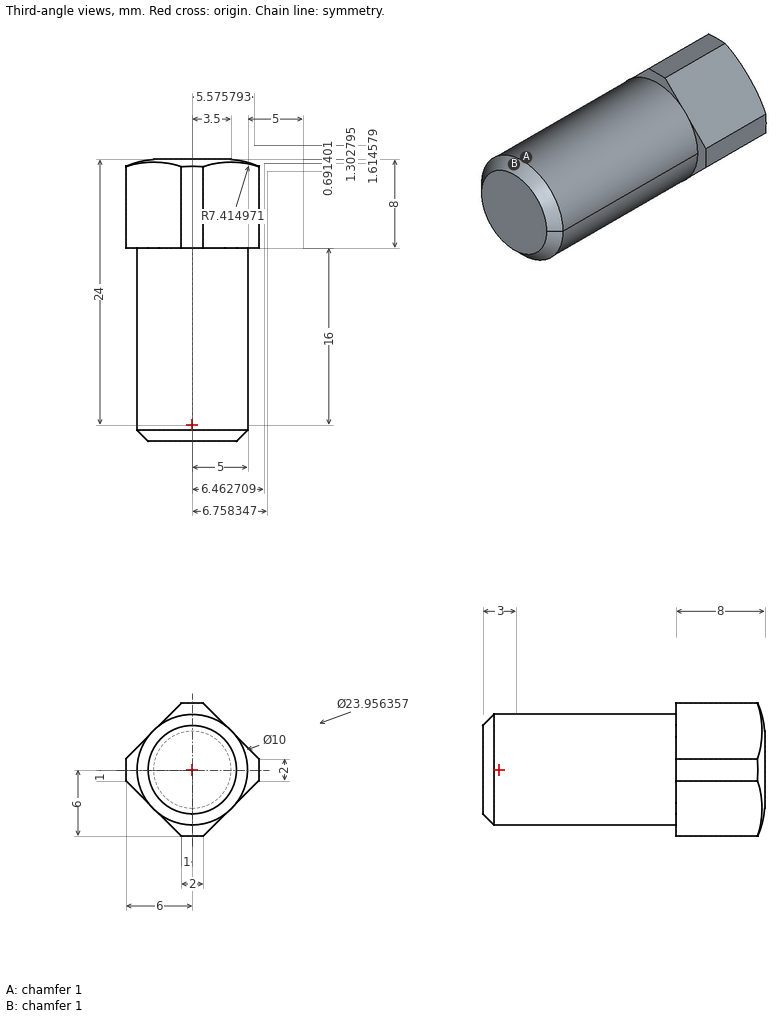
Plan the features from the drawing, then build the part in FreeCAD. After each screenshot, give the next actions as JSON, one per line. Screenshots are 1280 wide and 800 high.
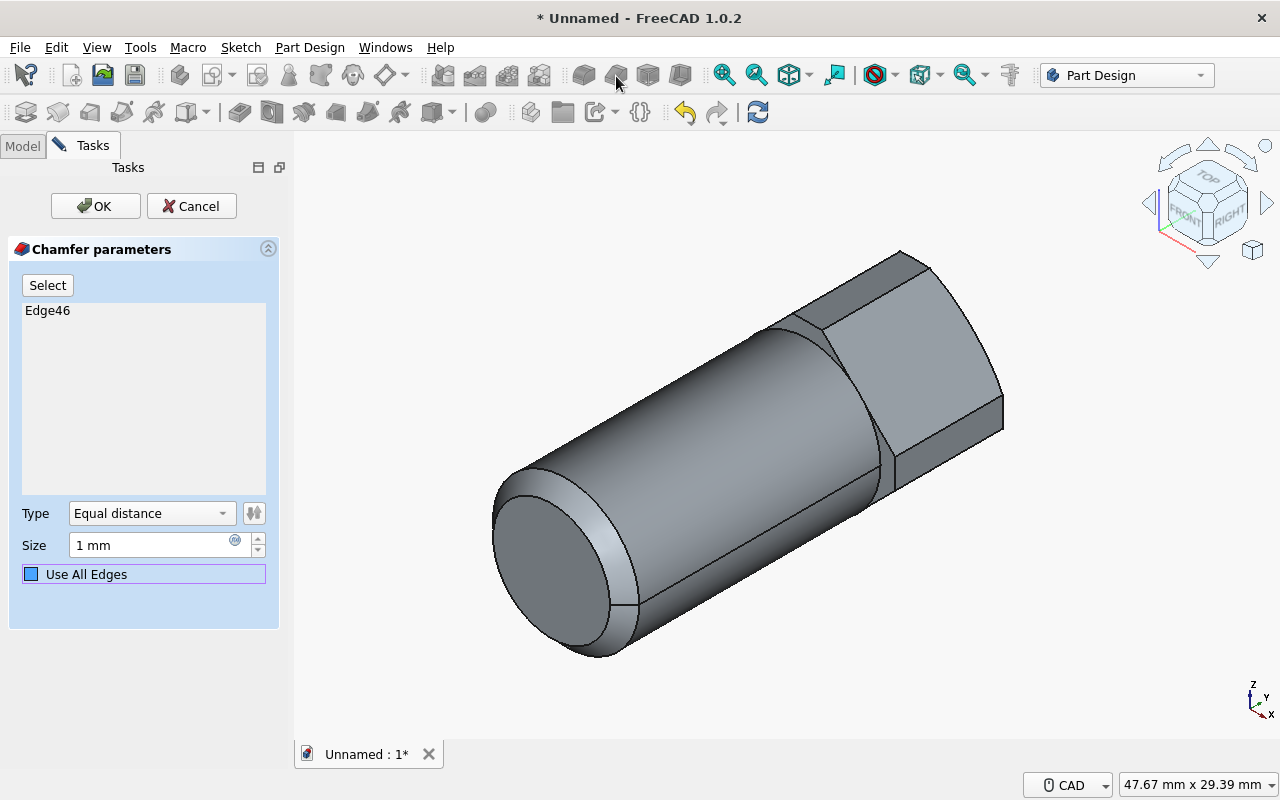
{"action": "left_click", "coordinate": [96, 206]}